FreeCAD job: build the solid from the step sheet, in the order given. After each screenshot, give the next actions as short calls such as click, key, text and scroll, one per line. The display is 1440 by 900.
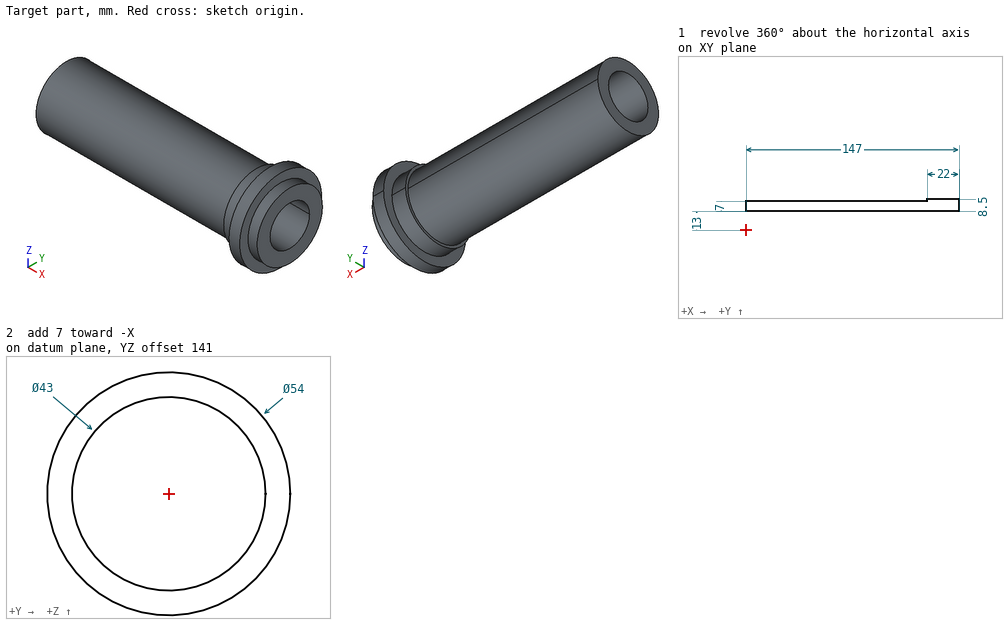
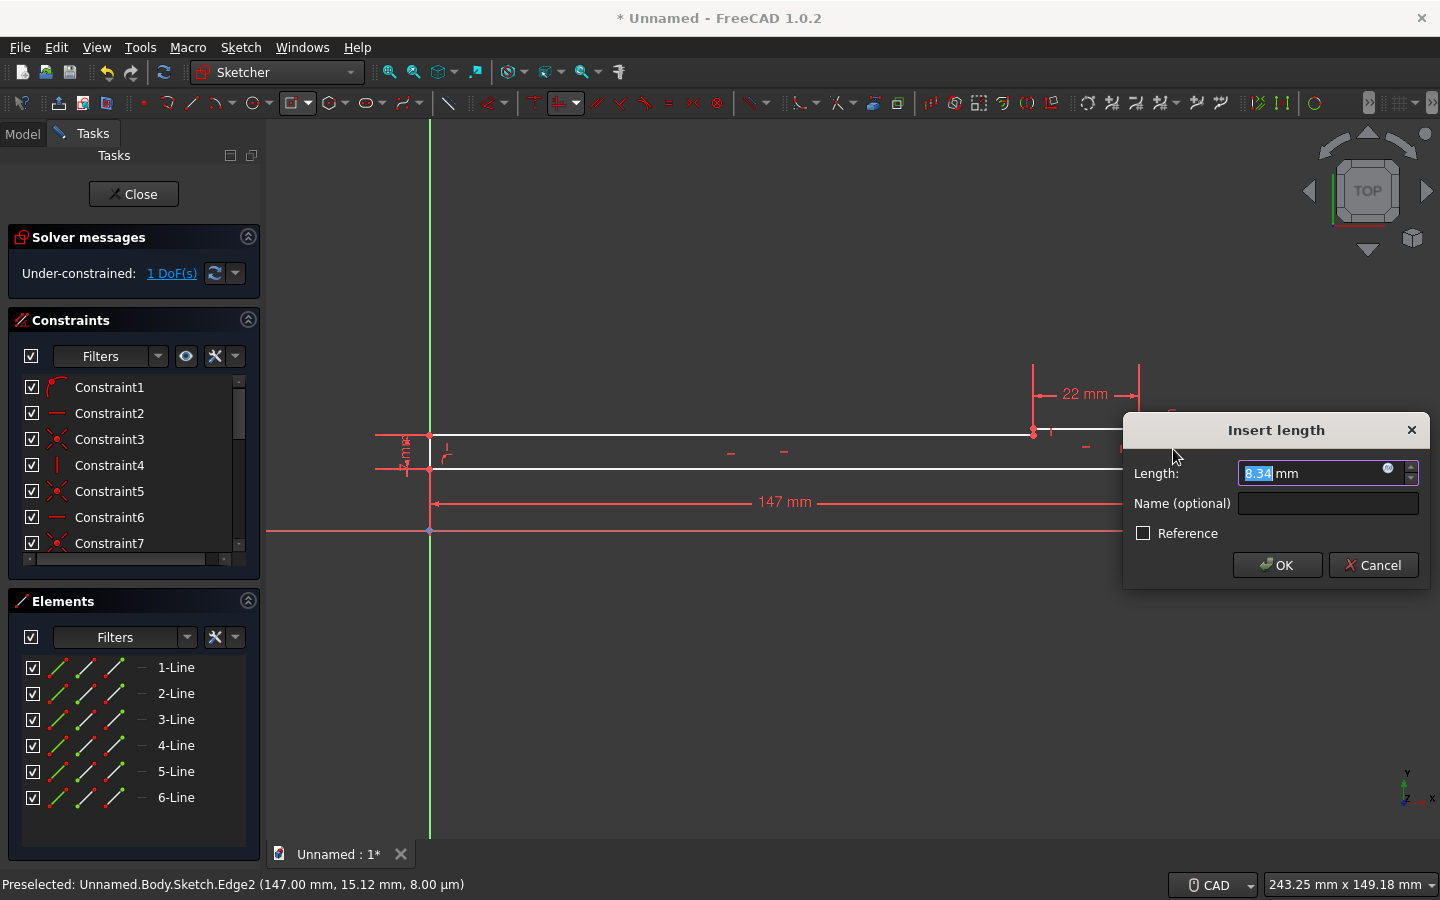
text(8.5)
key(Return)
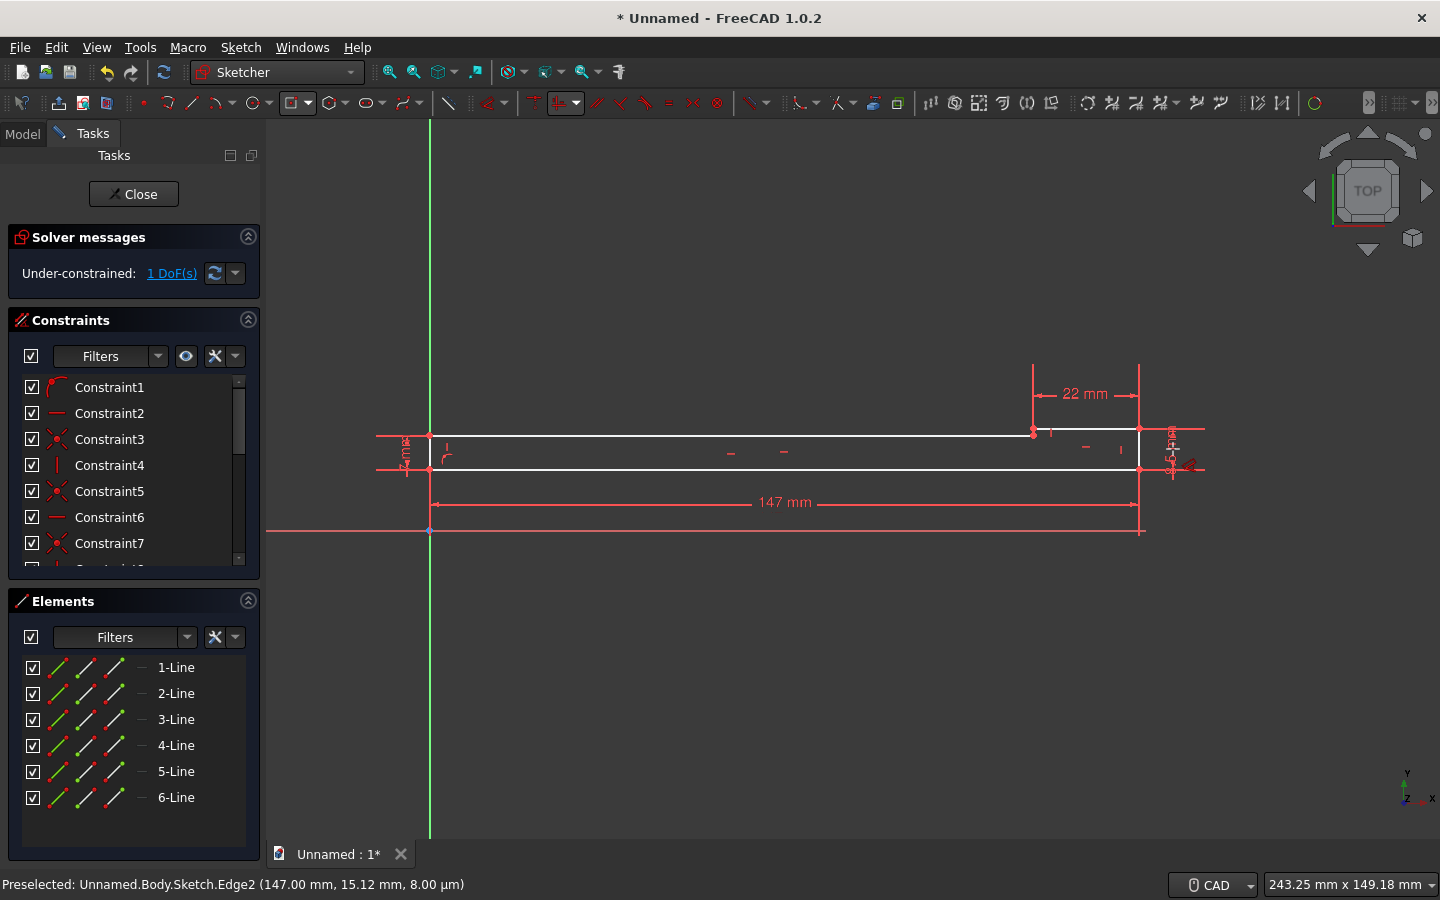
click(430, 470)
click(396, 500)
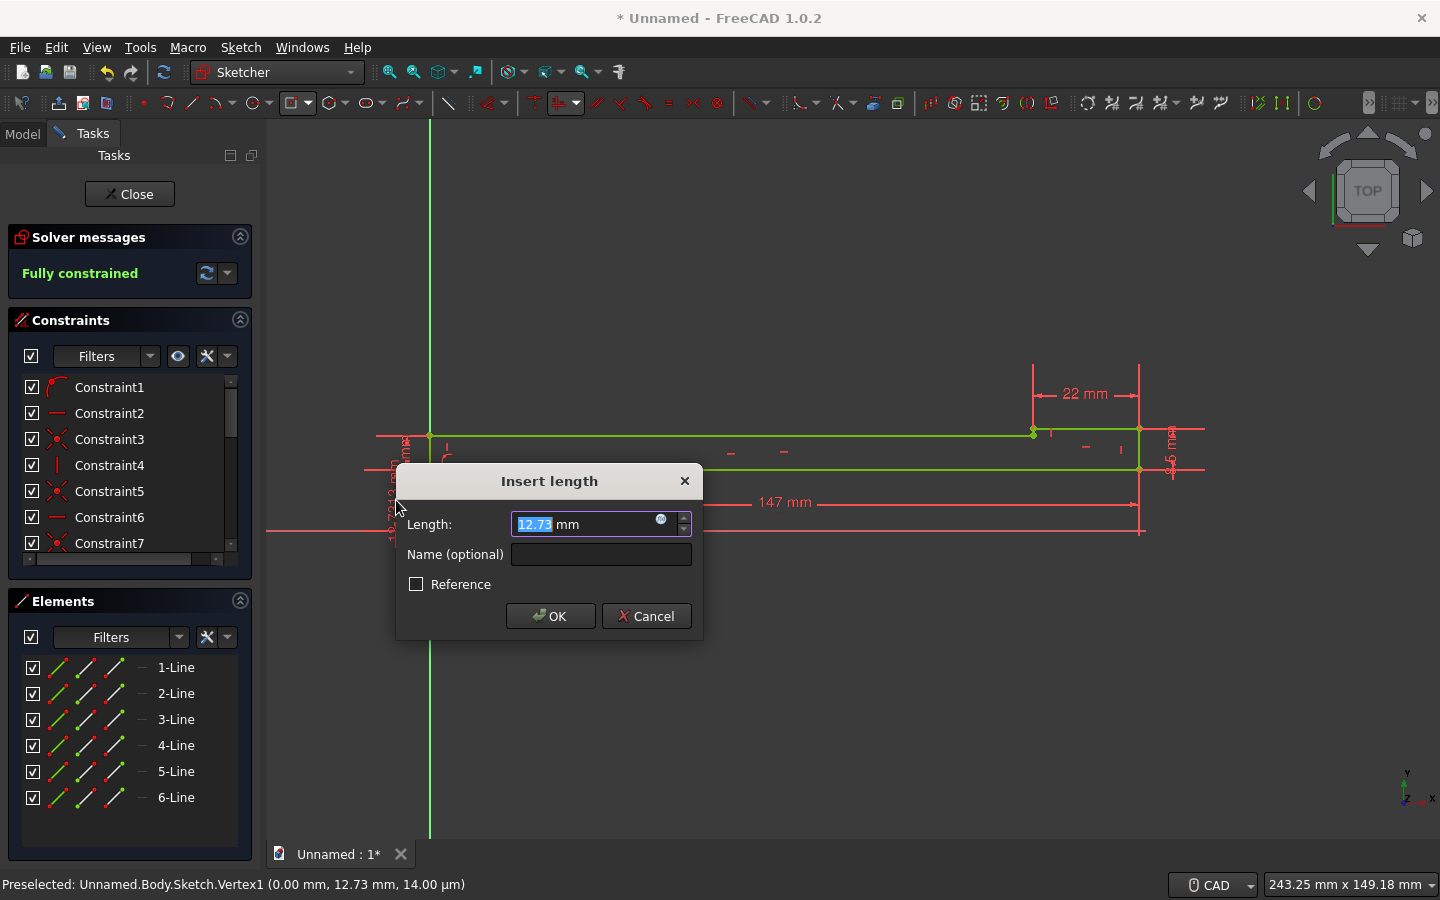
text(13)
key(Return)
key(Escape)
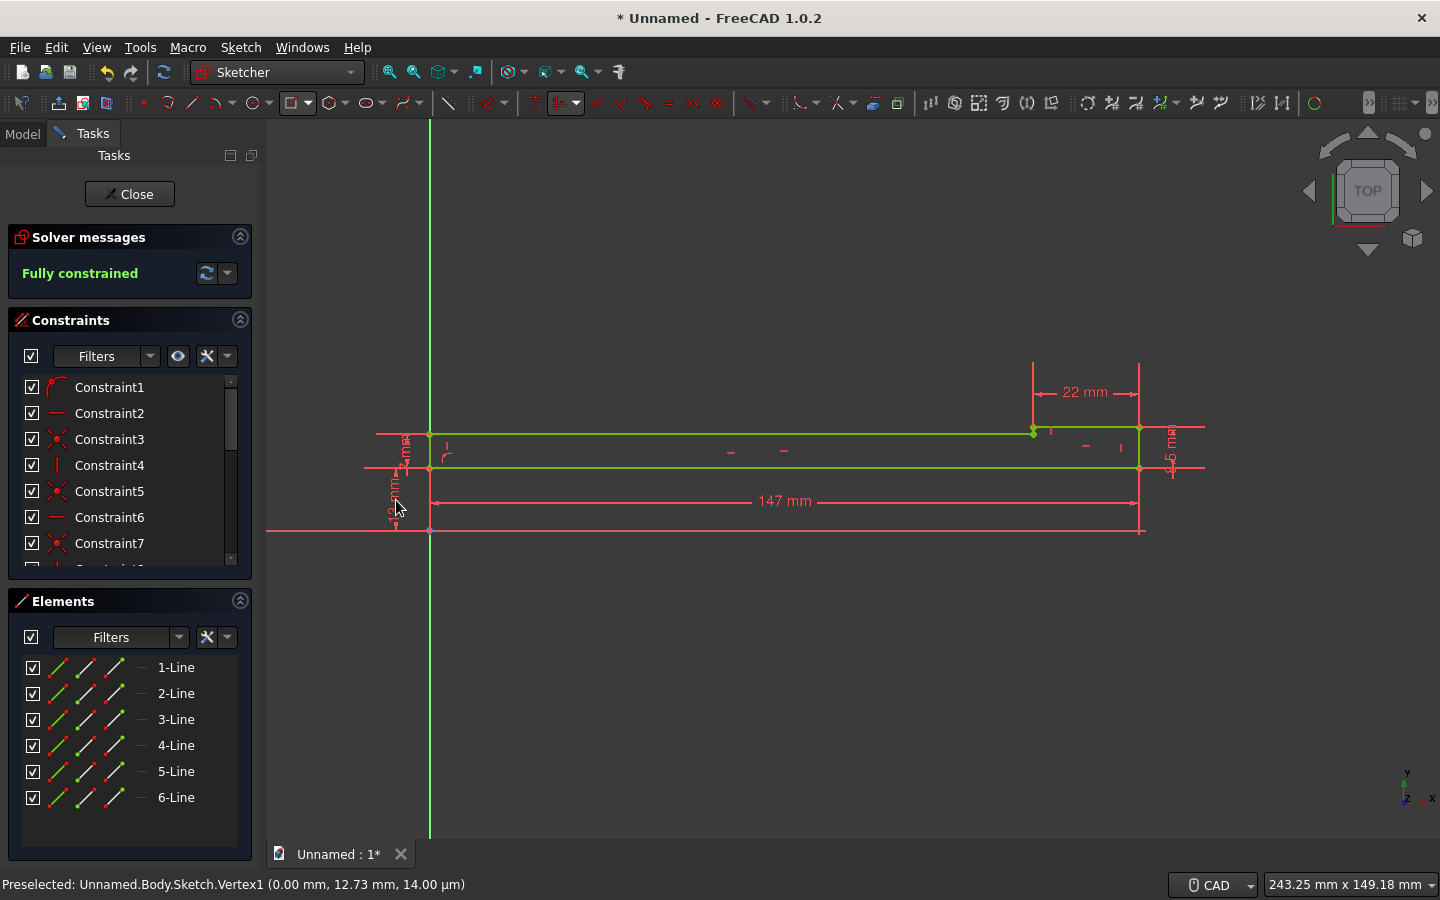
click(130, 194)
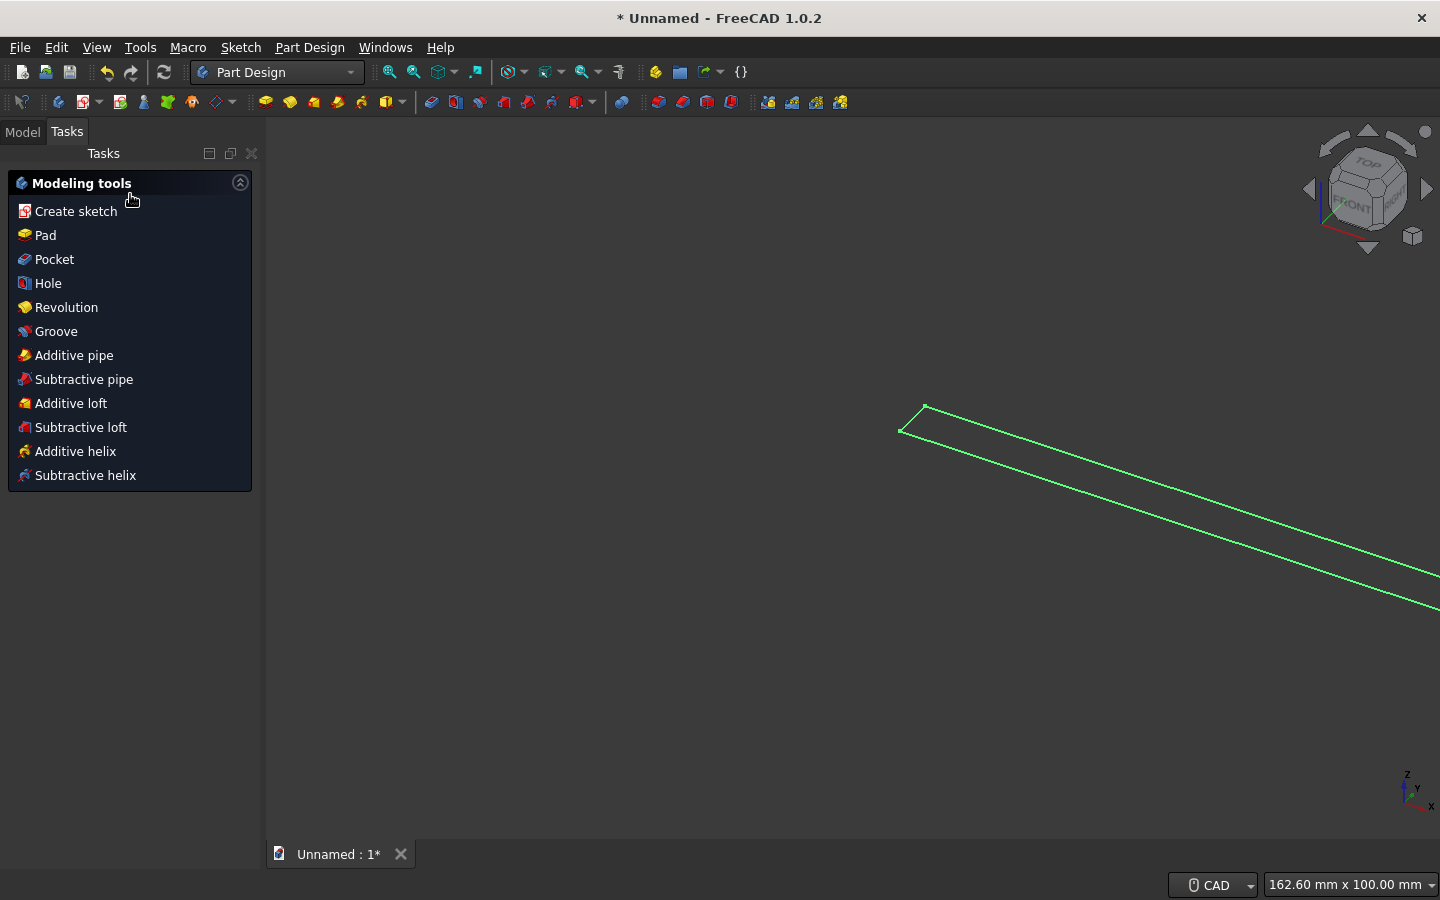
click(290, 102)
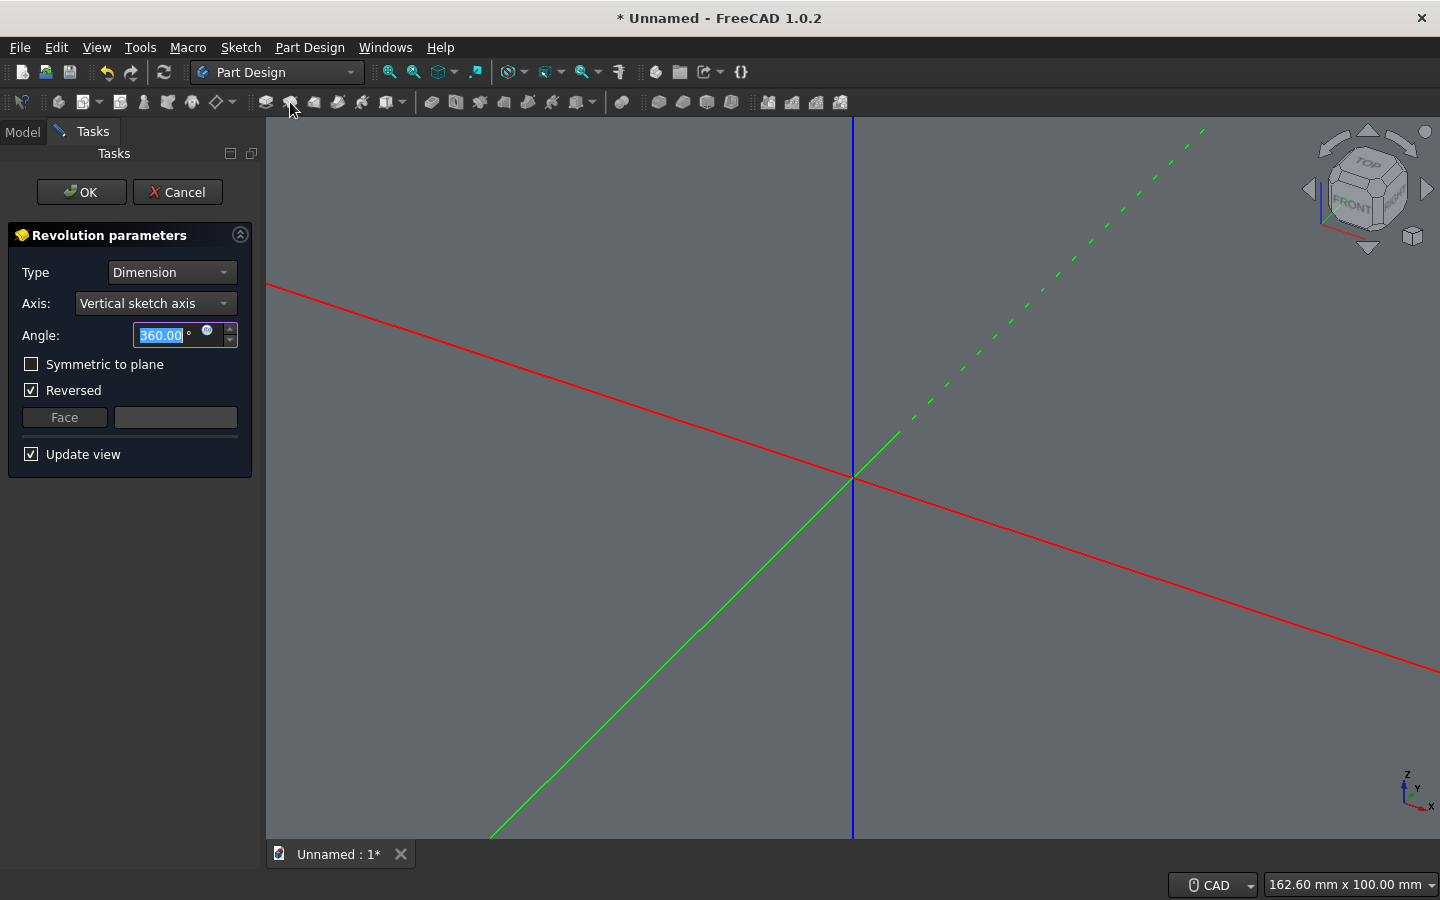
click(156, 304)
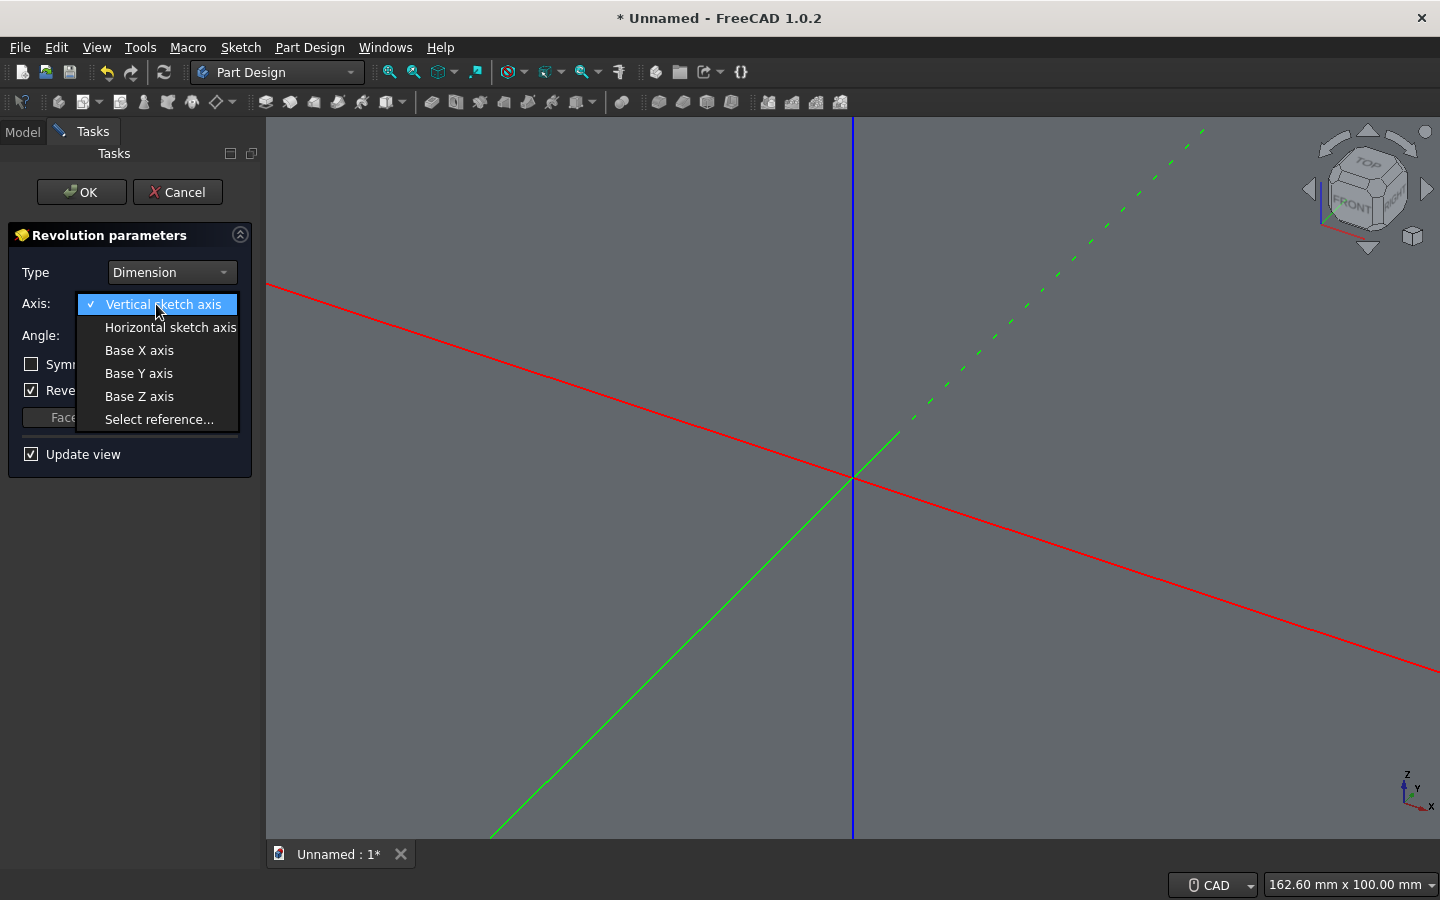
click(156, 328)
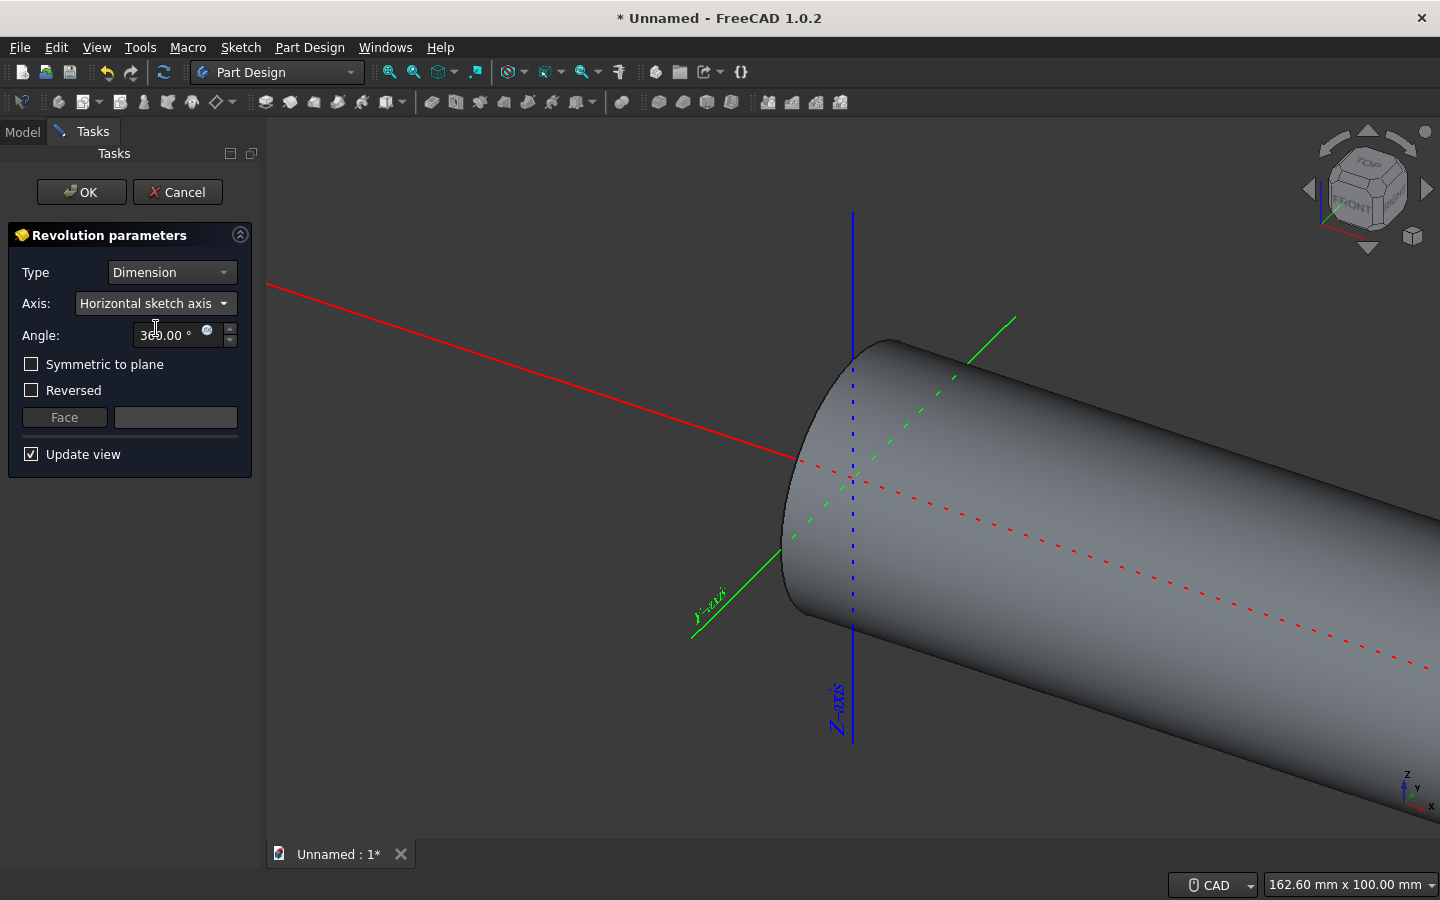
click(82, 192)